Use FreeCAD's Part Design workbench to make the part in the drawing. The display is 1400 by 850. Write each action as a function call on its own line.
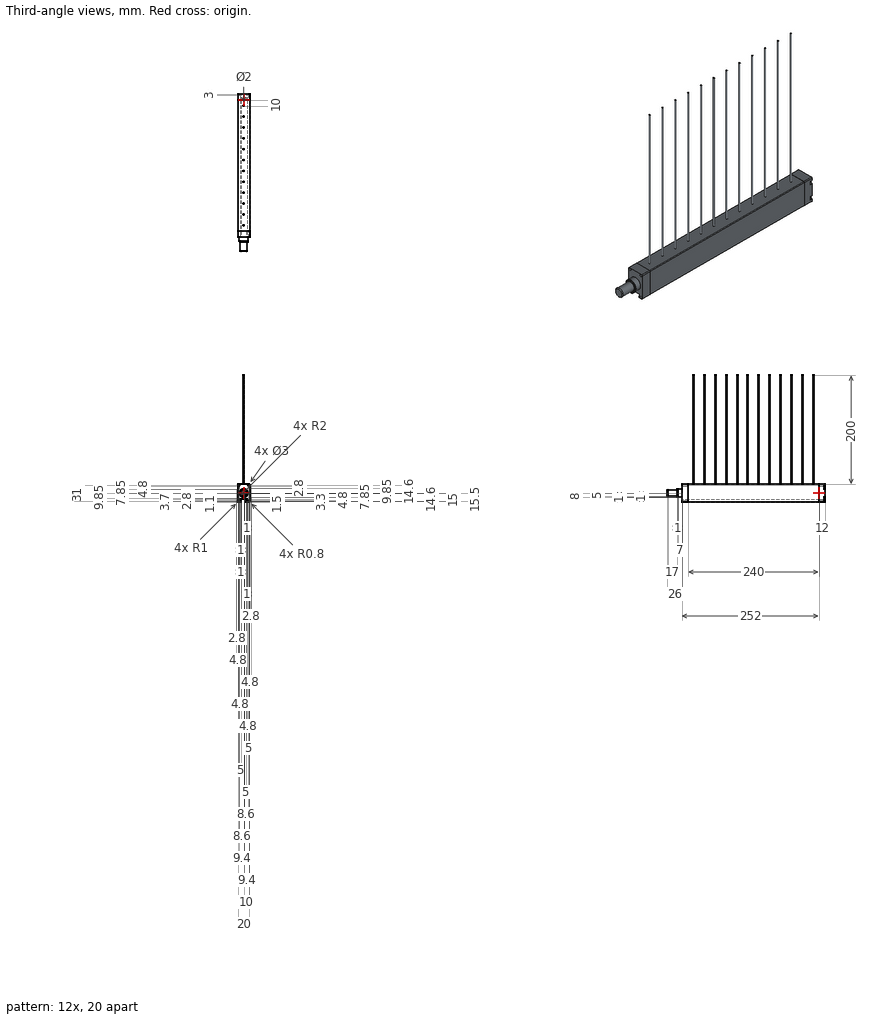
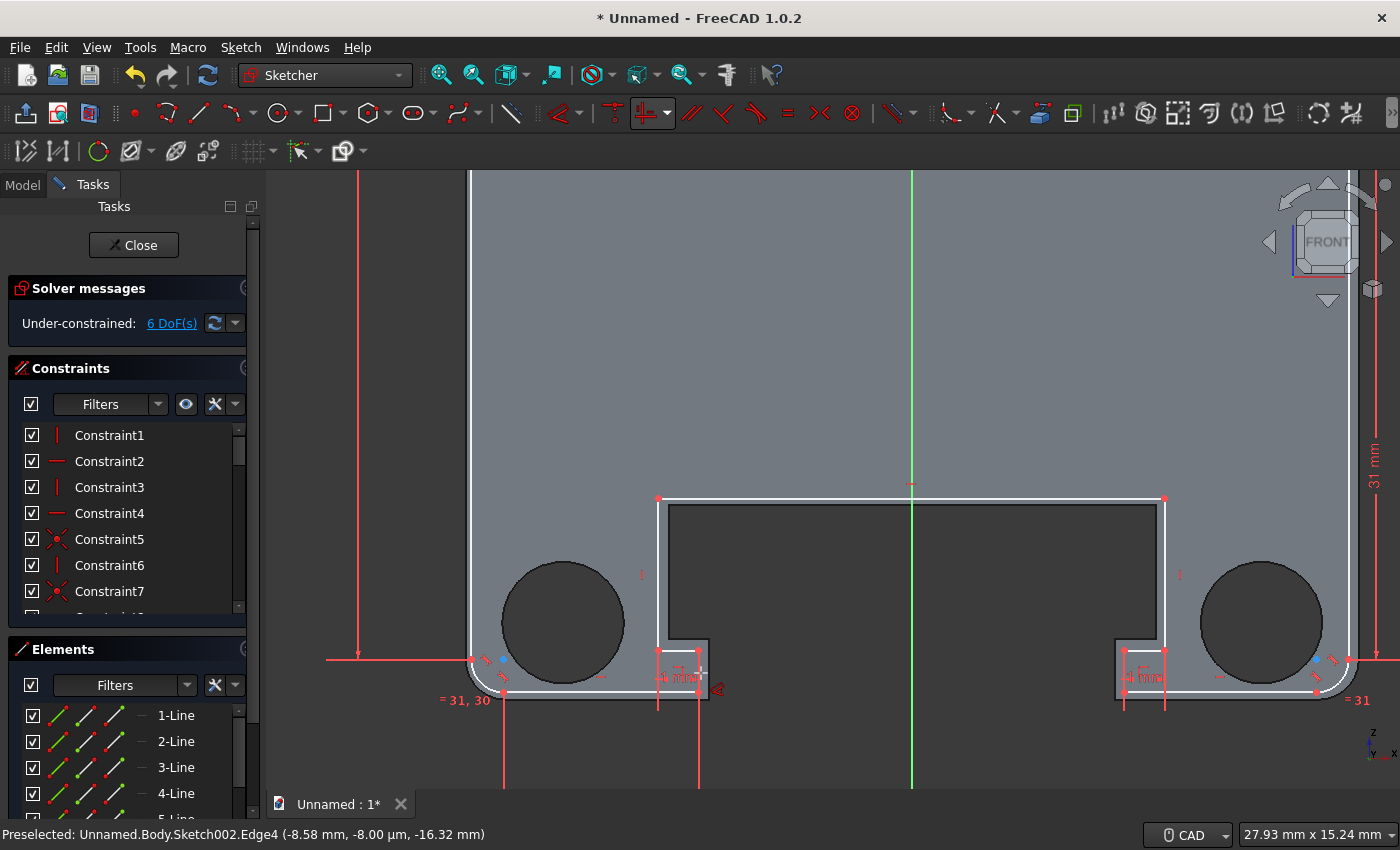
click(699, 672)
click(733, 657)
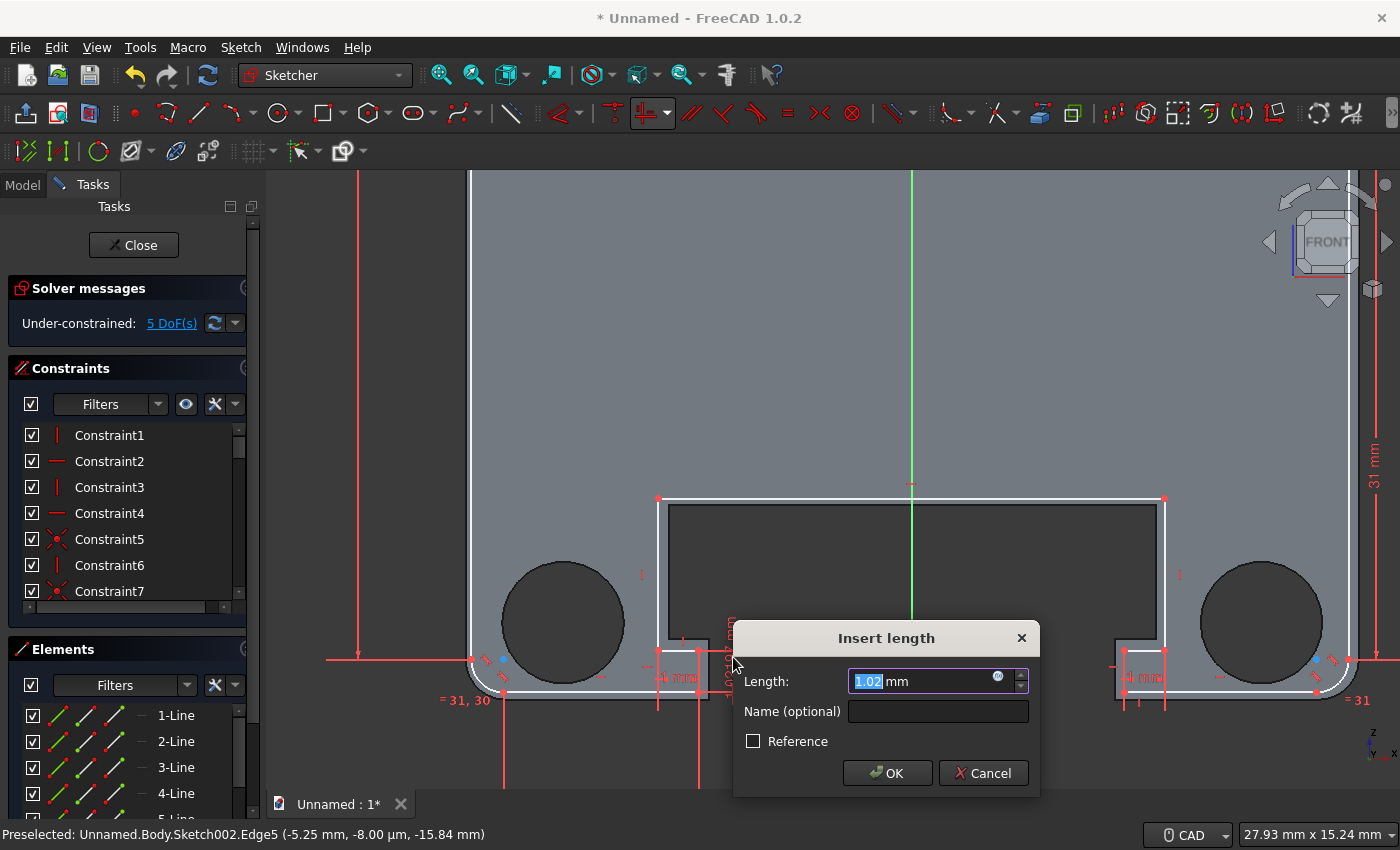
text(1.1)
key(Return)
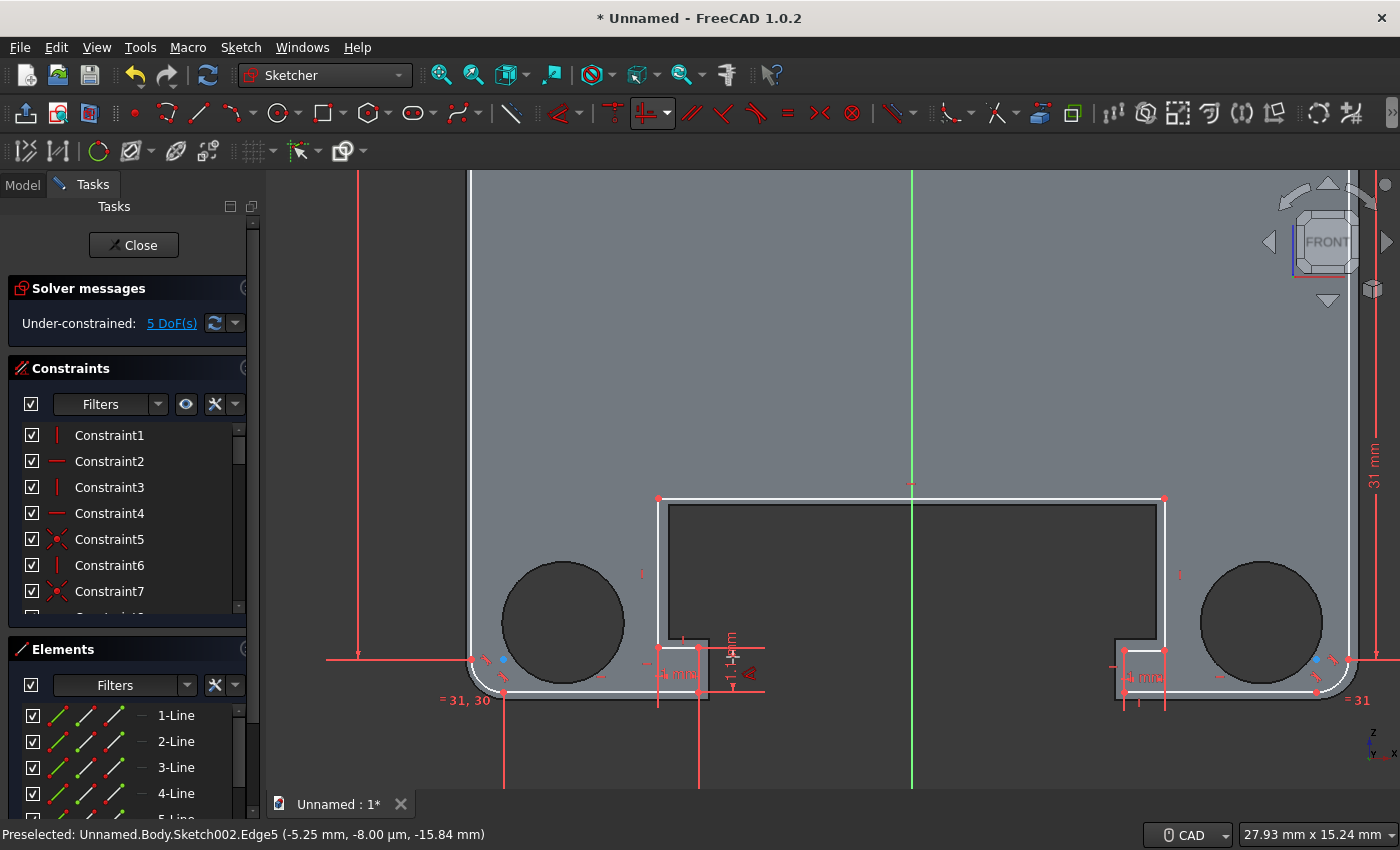
click(658, 603)
click(624, 573)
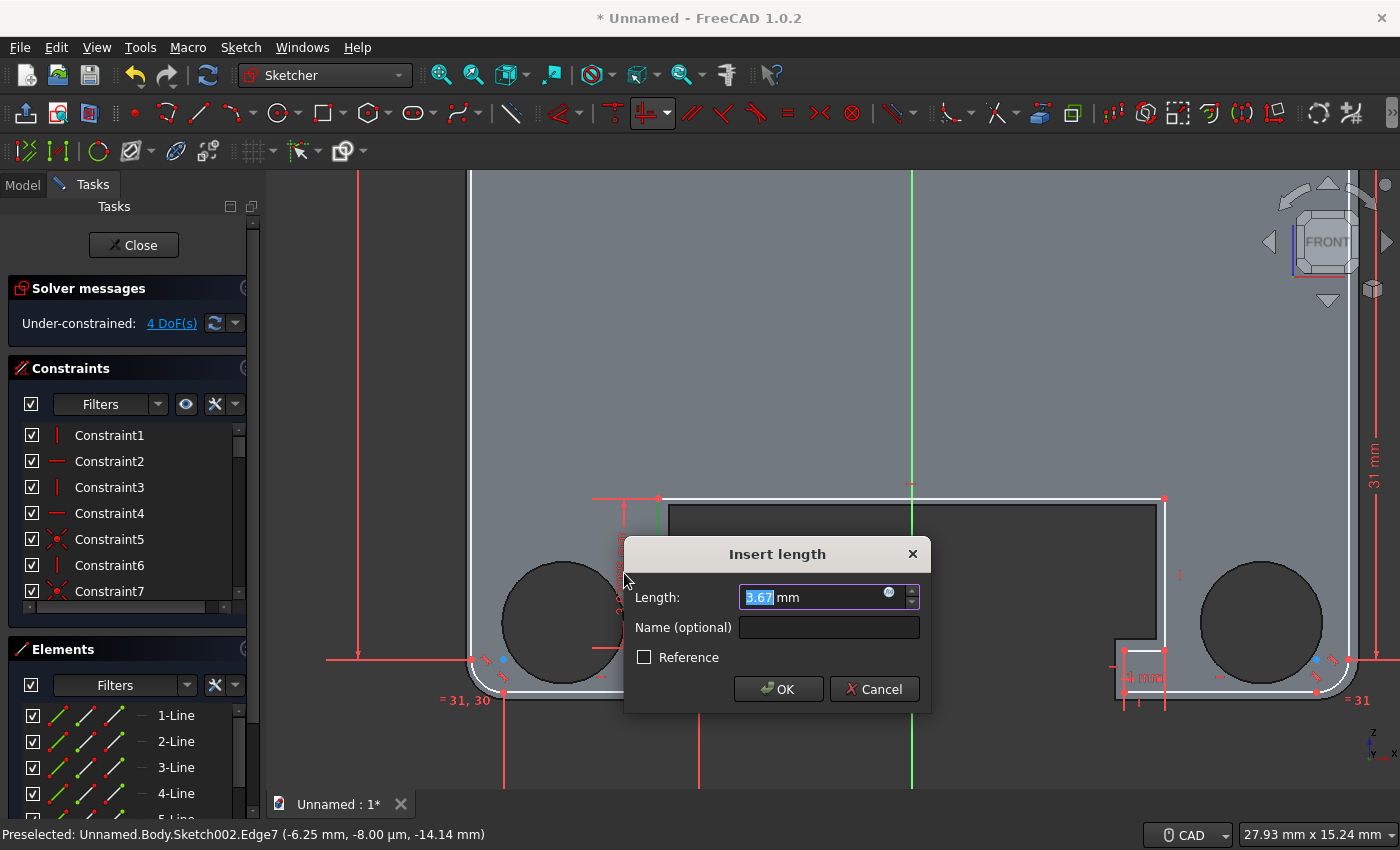
text(3.7)
key(Return)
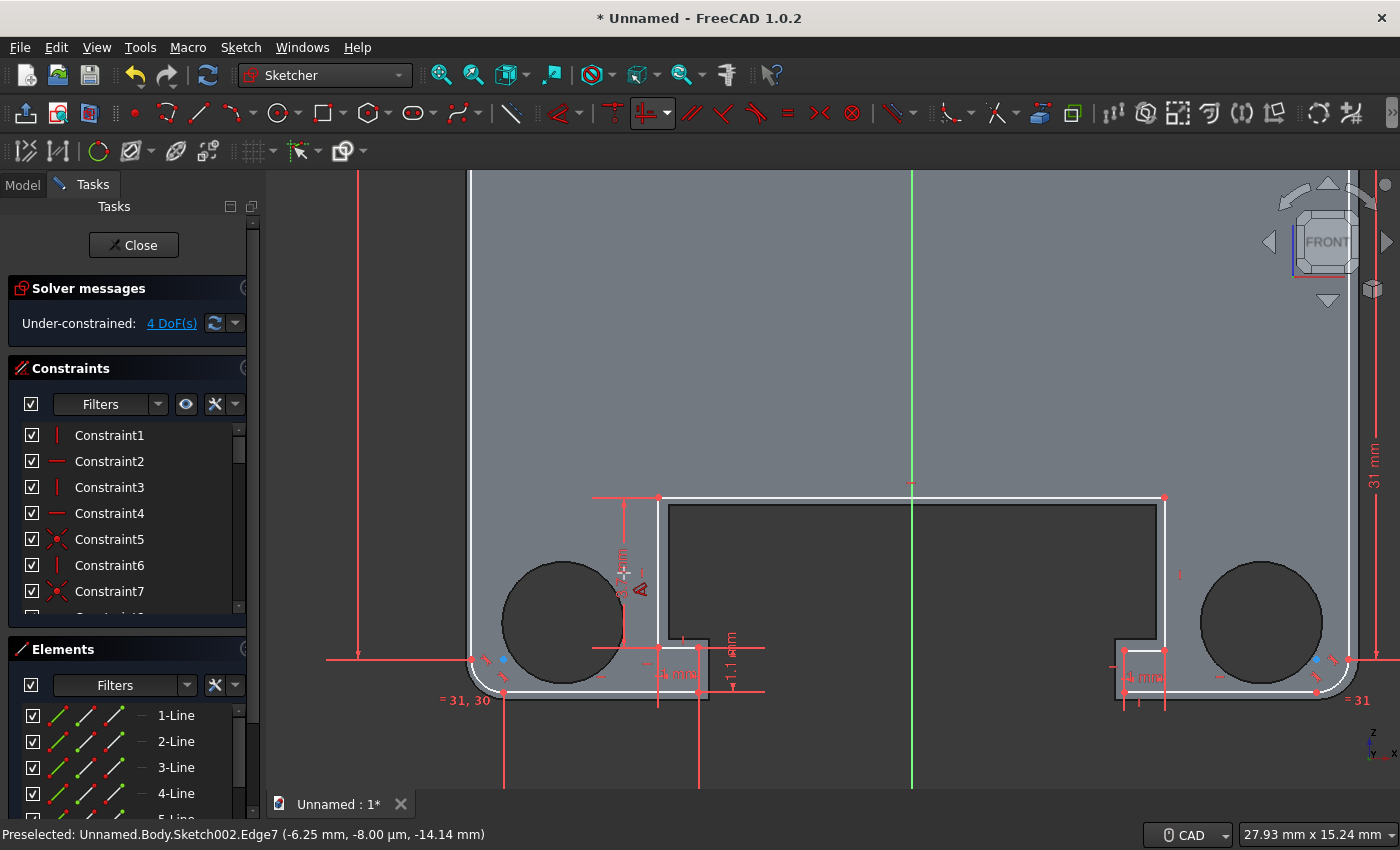
click(1165, 544)
click(1199, 574)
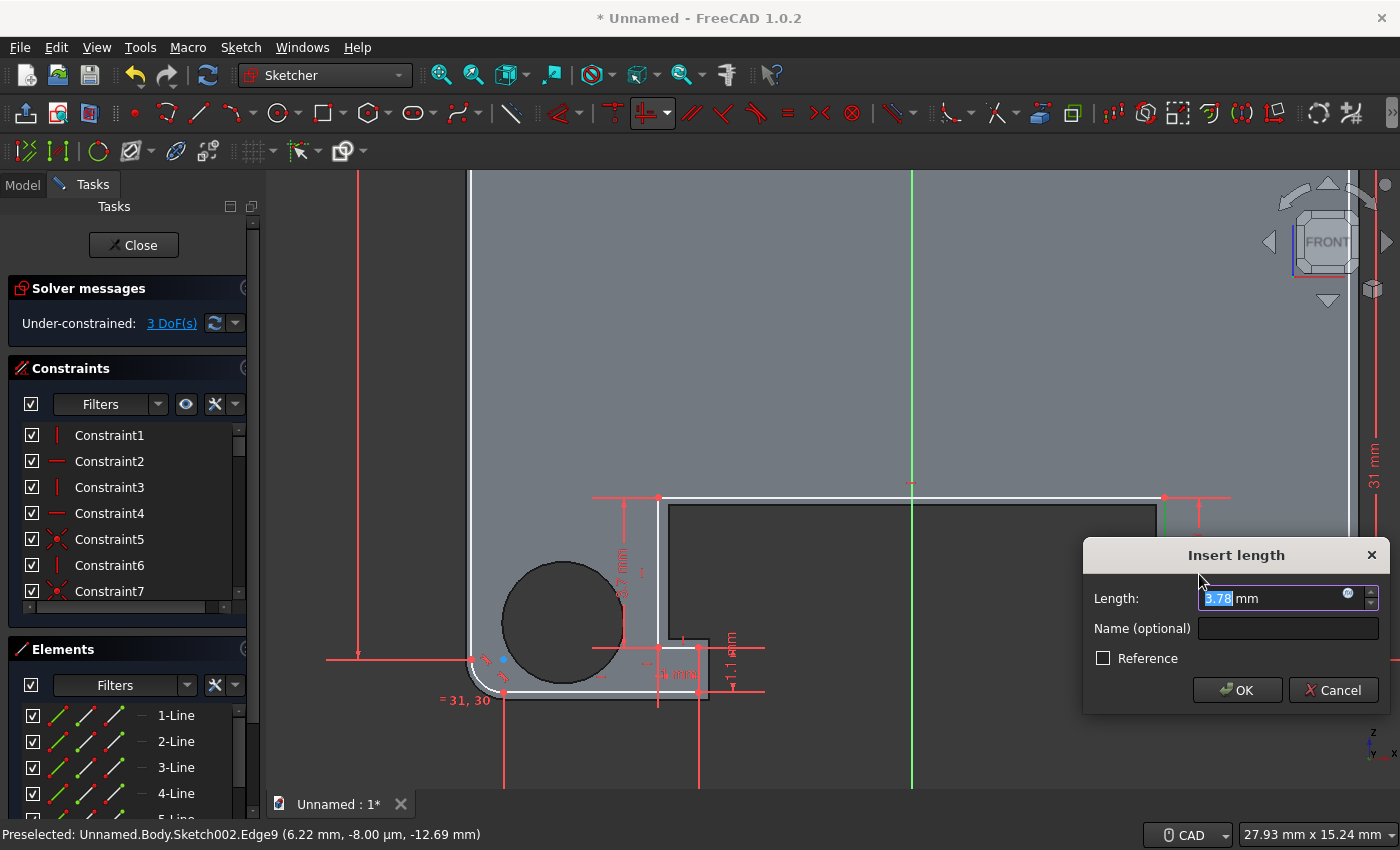
text(3.7)
key(Return)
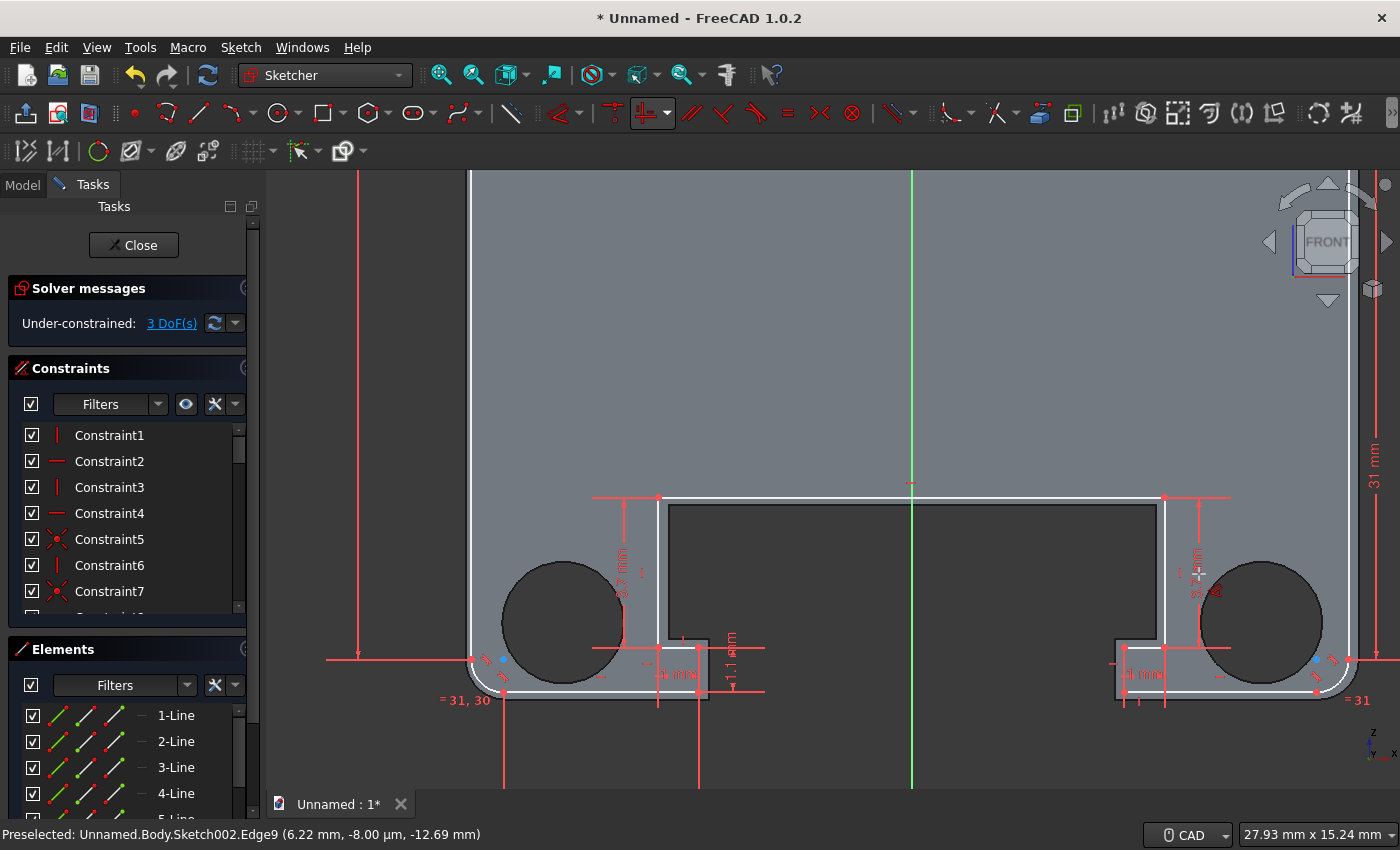
click(1182, 692)
click(1180, 726)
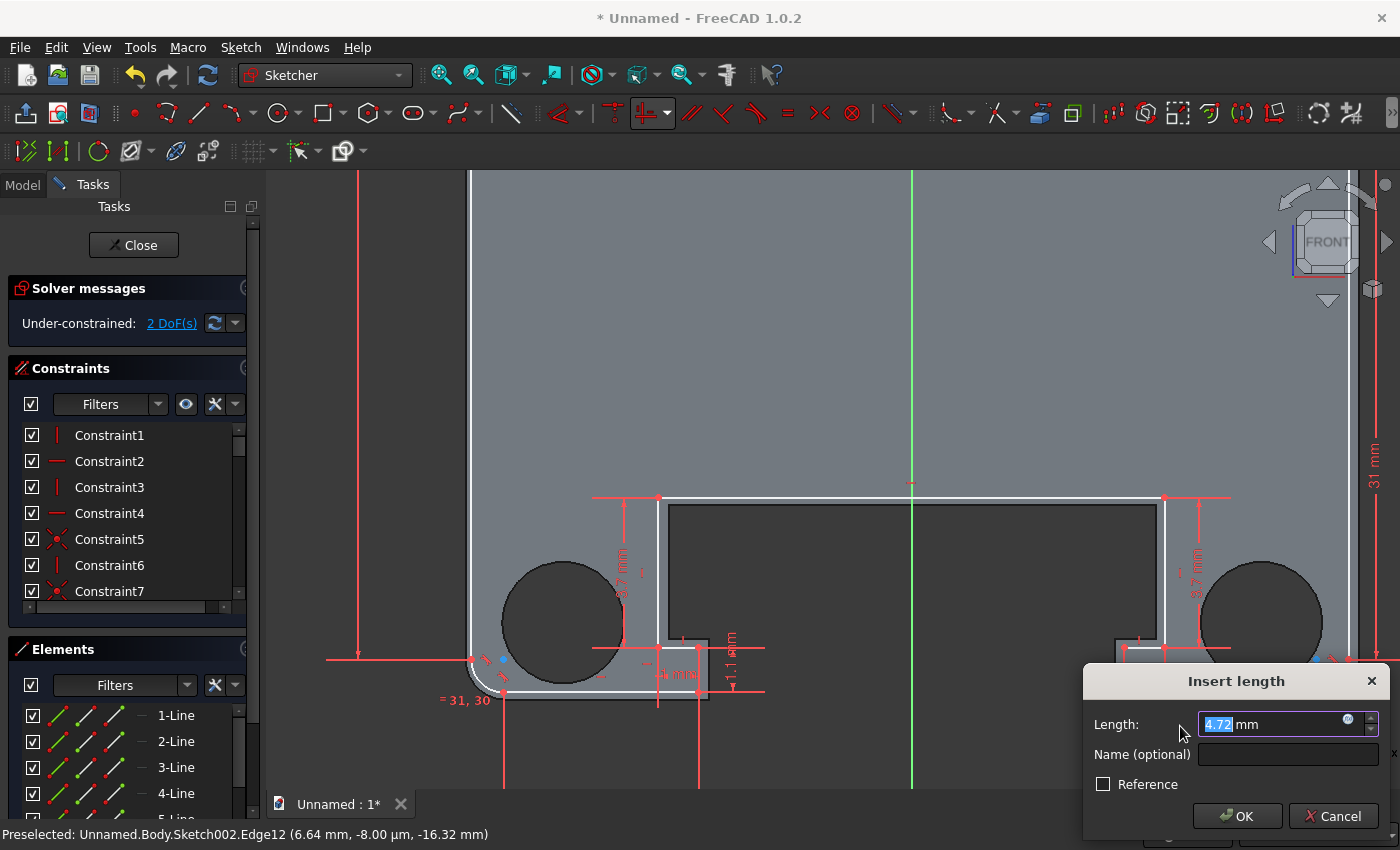
text(4.8)
key(Return)